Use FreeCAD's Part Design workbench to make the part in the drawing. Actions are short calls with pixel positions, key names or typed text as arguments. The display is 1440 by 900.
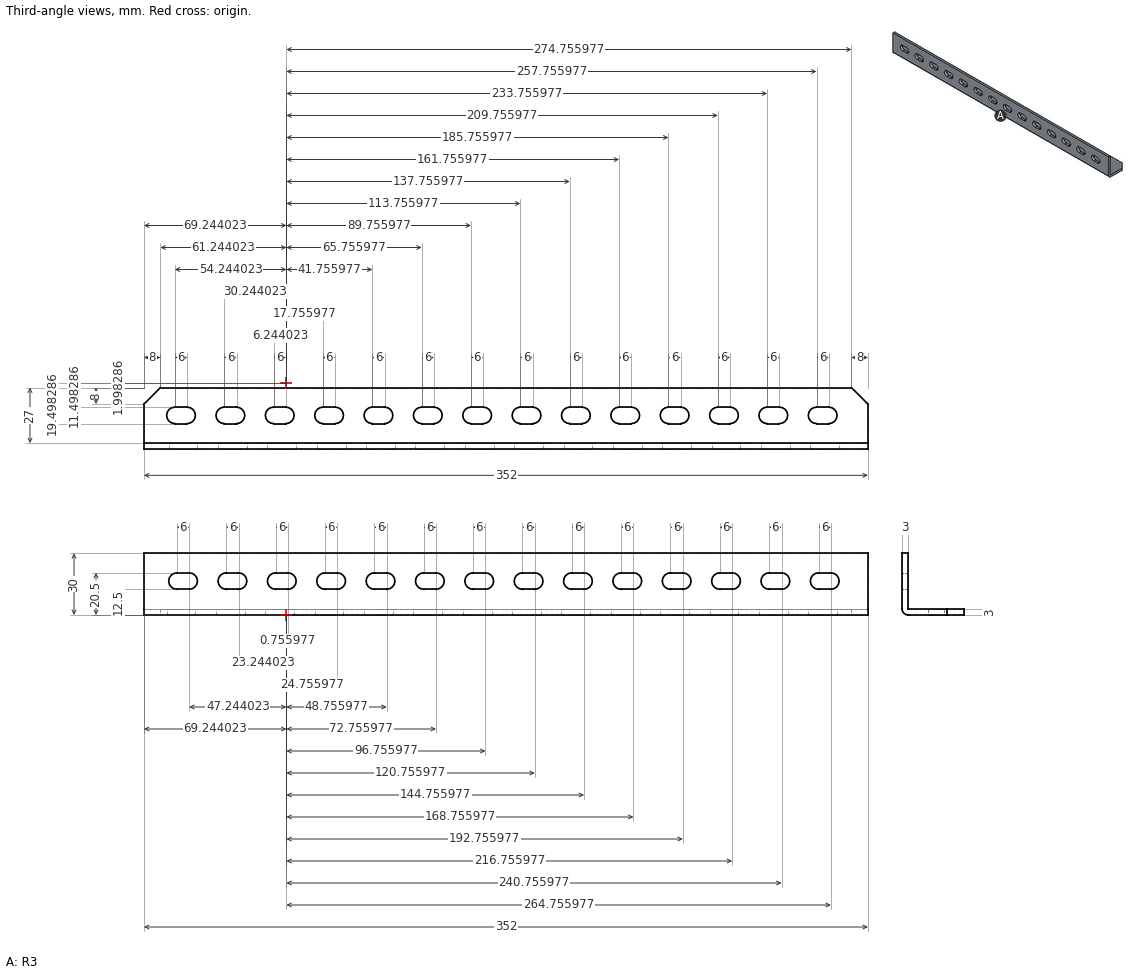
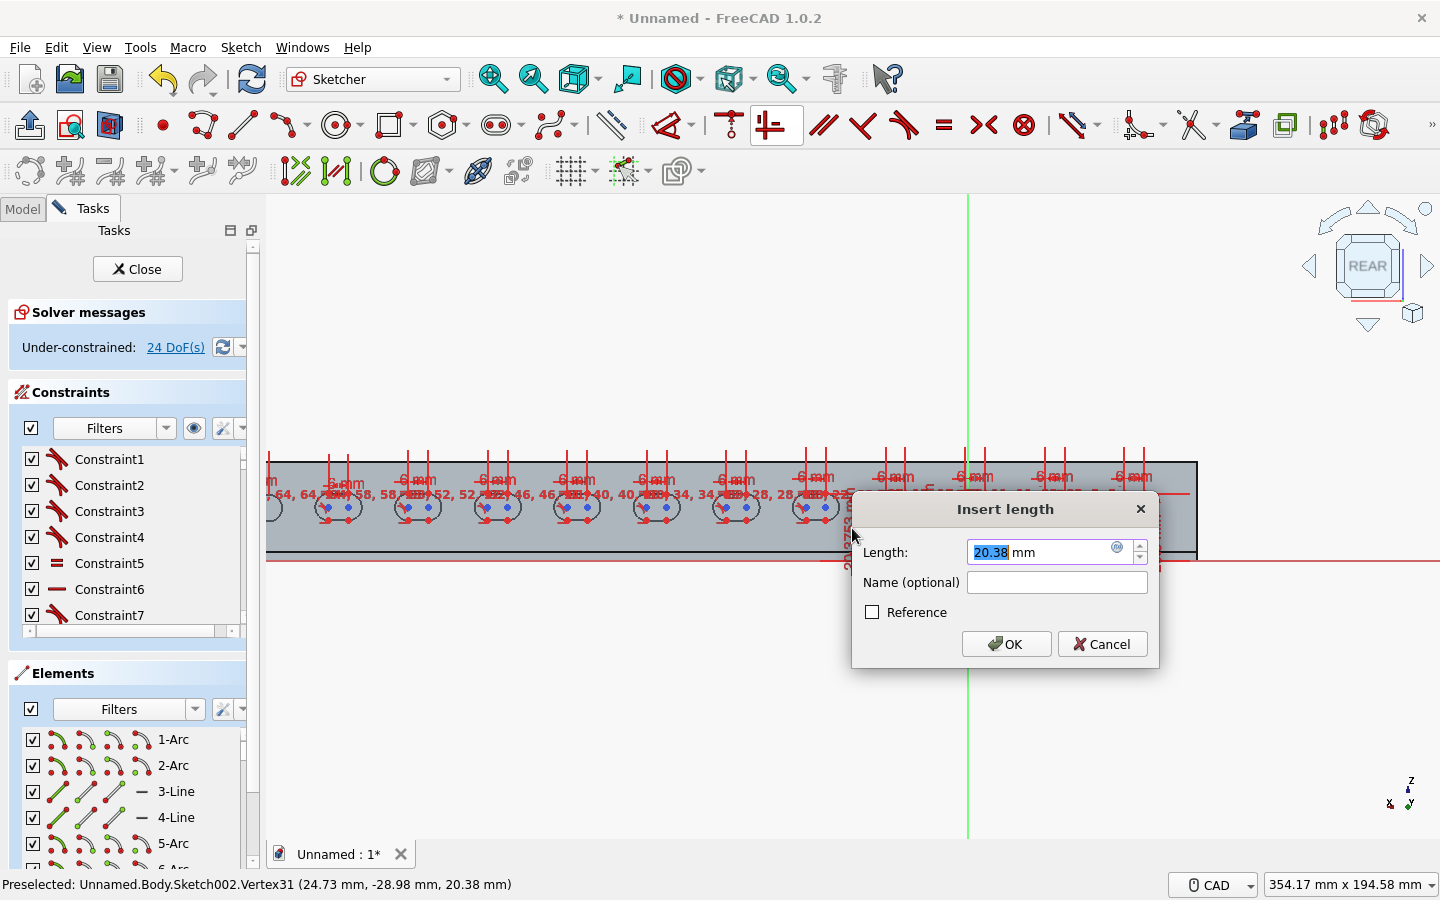
text(20.5)
key(Return)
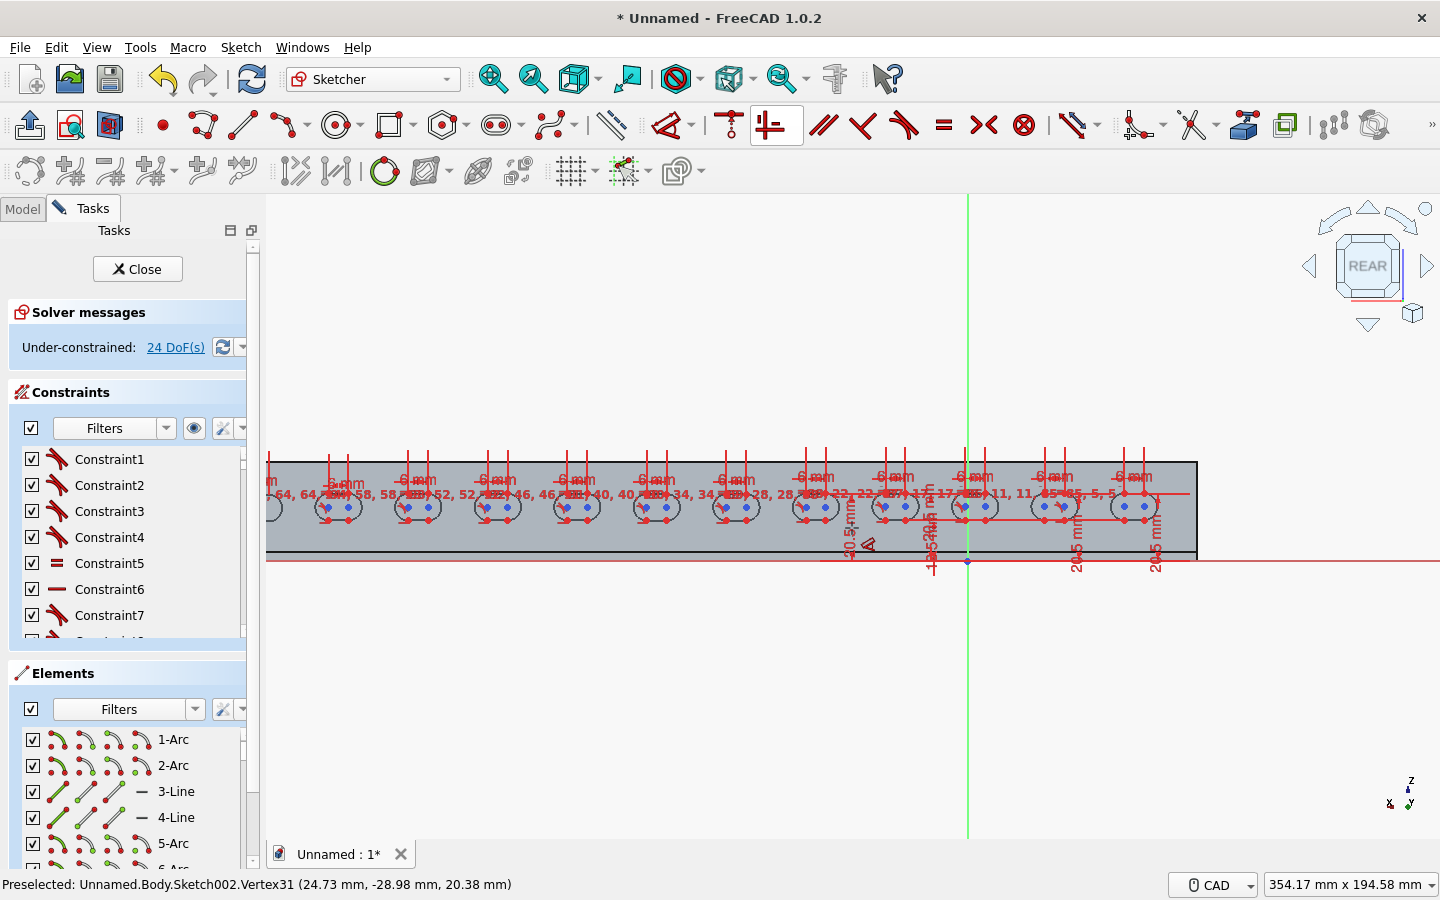
click(806, 494)
click(772, 528)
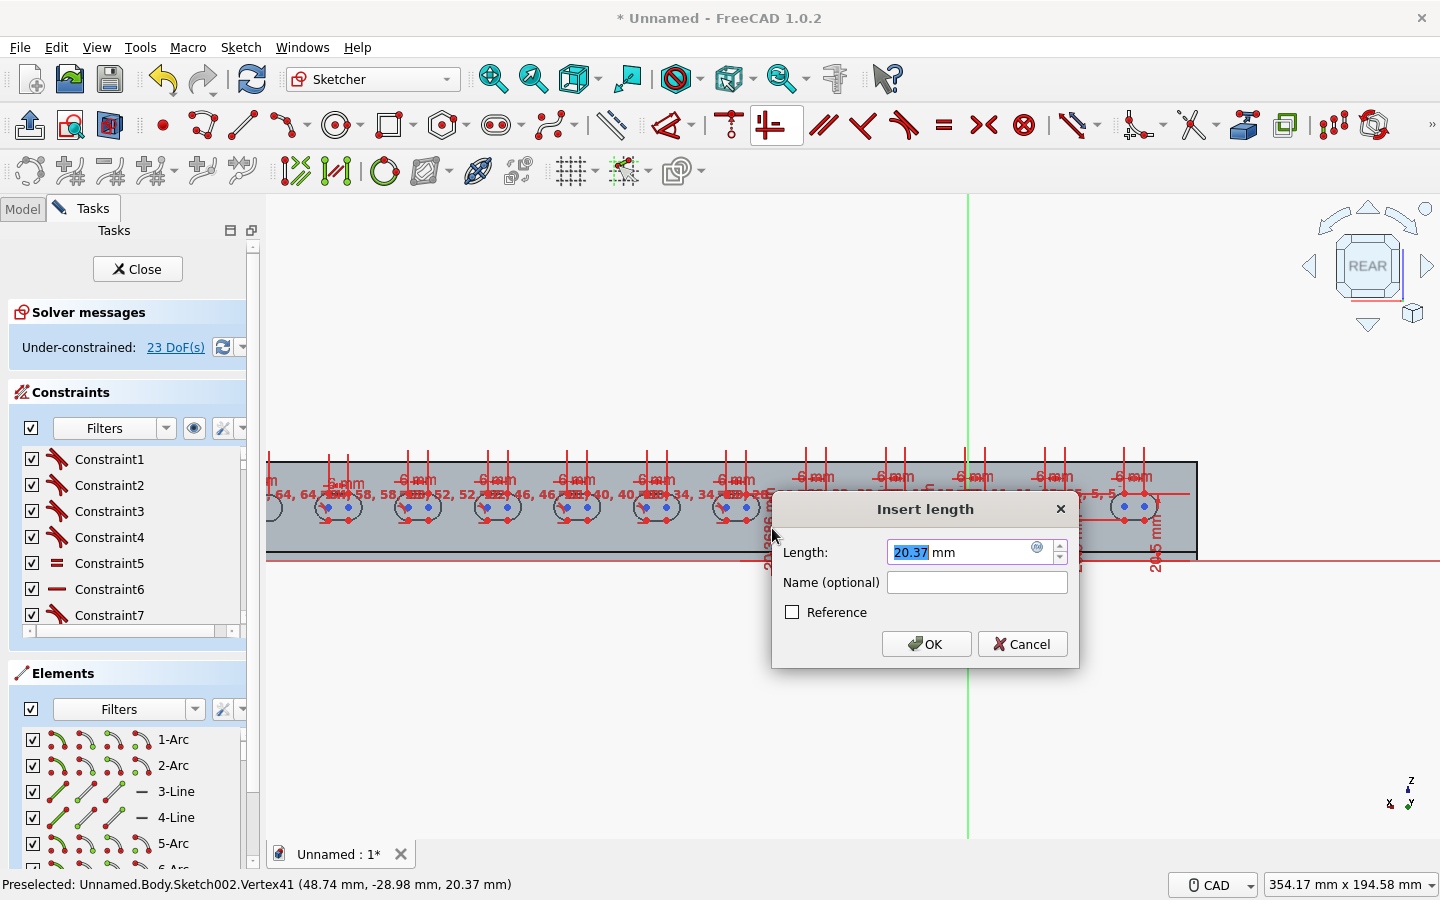
text(20.5)
key(Return)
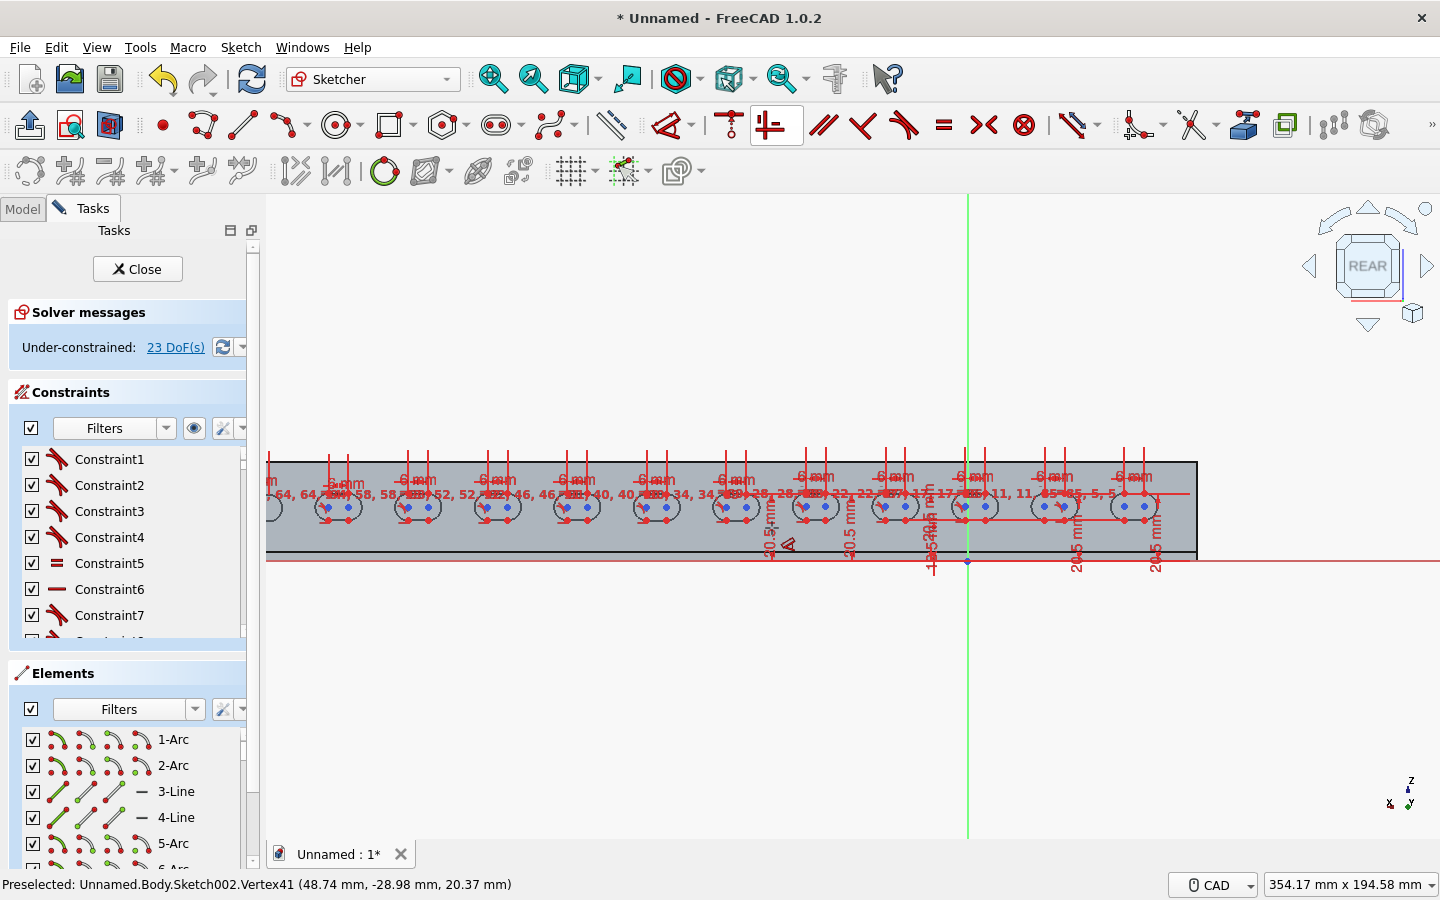
click(726, 494)
click(692, 528)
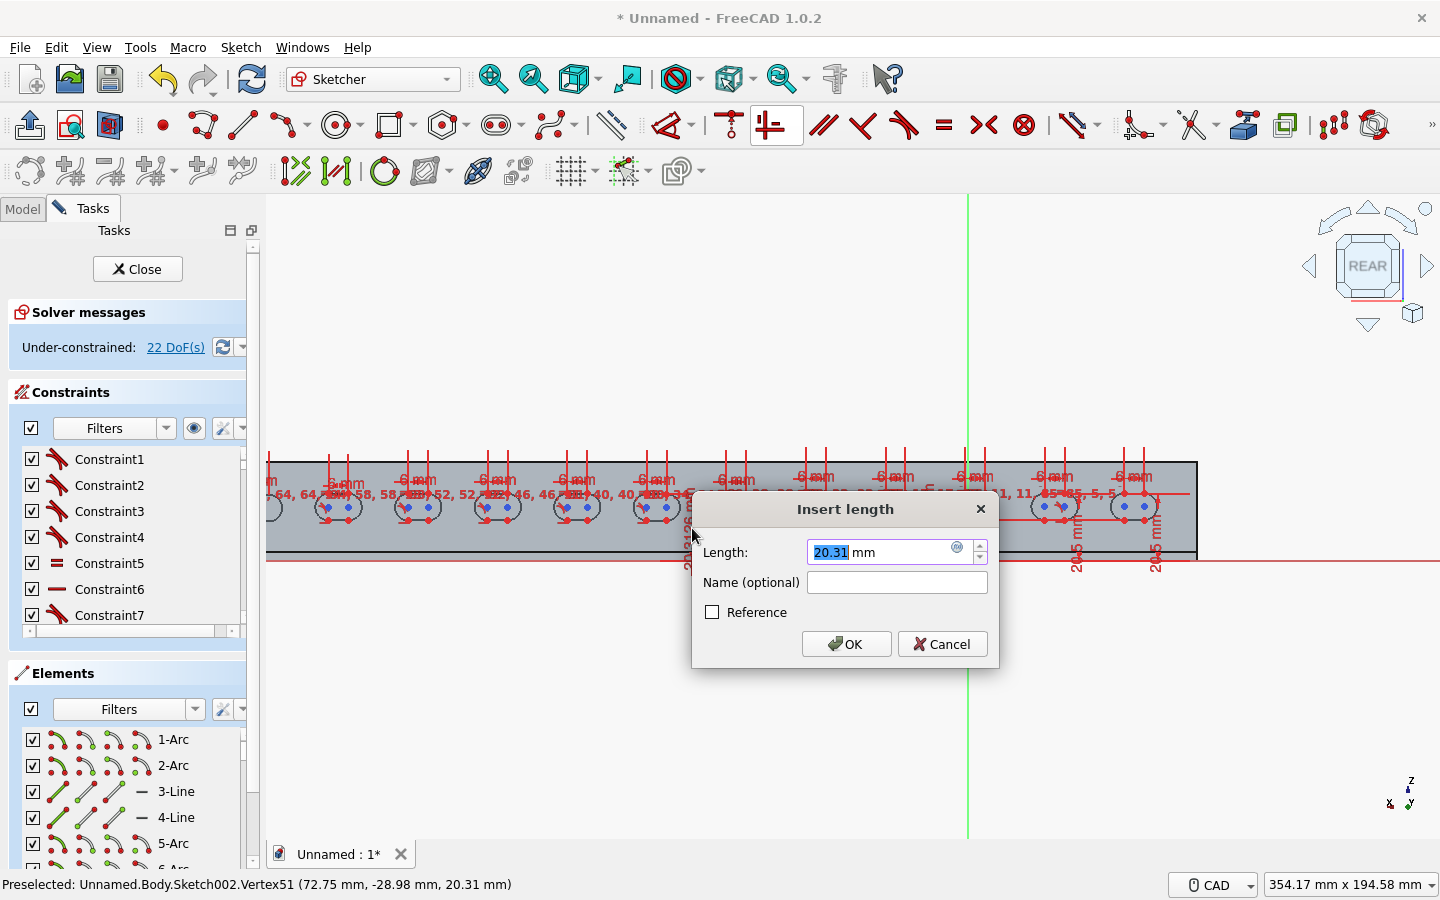
text(20.5)
key(Return)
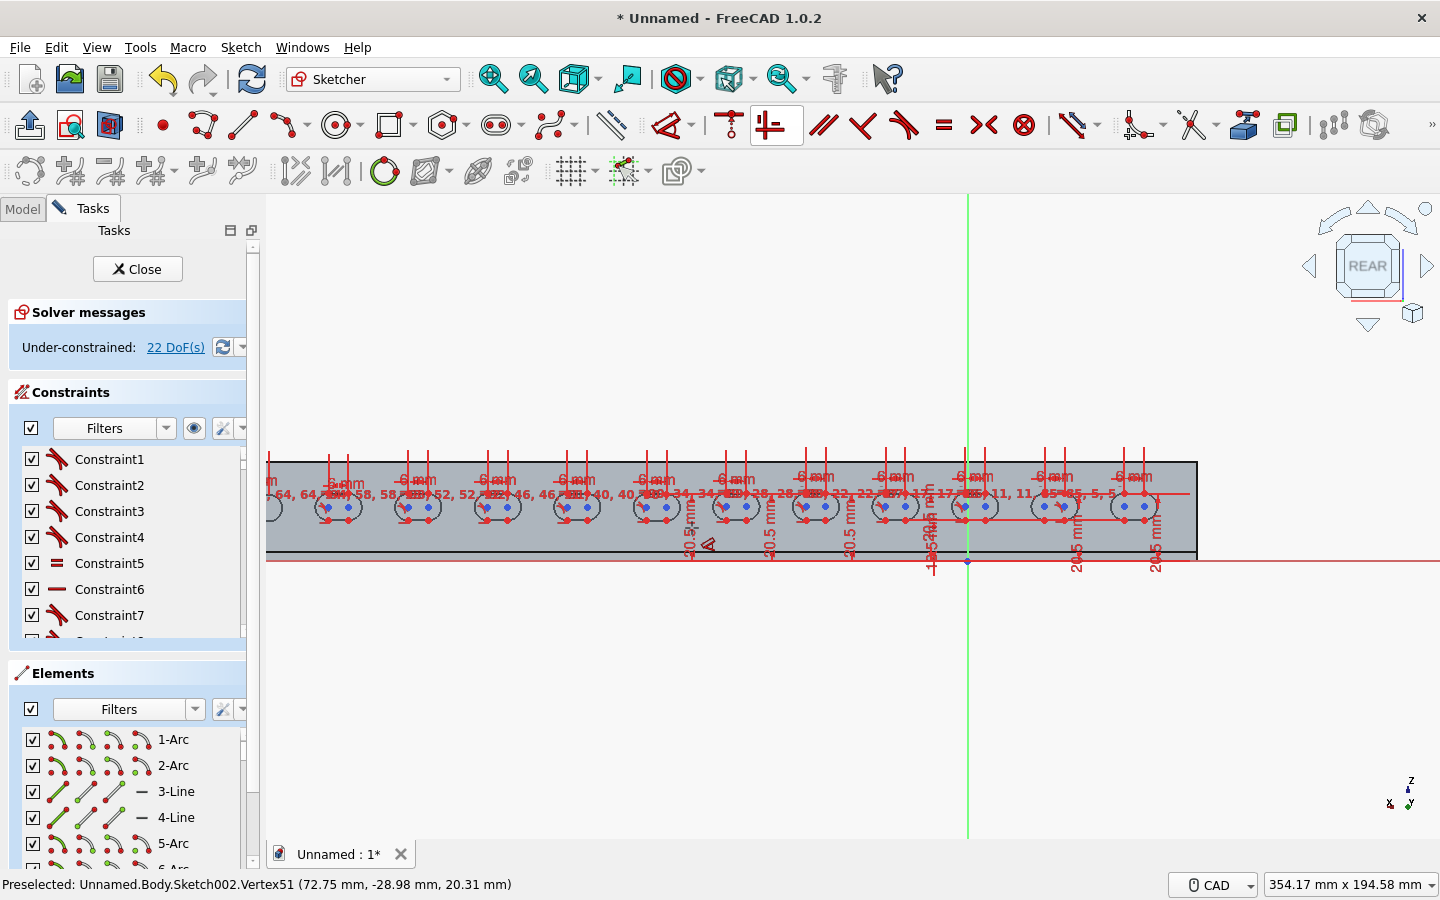
click(647, 494)
click(613, 528)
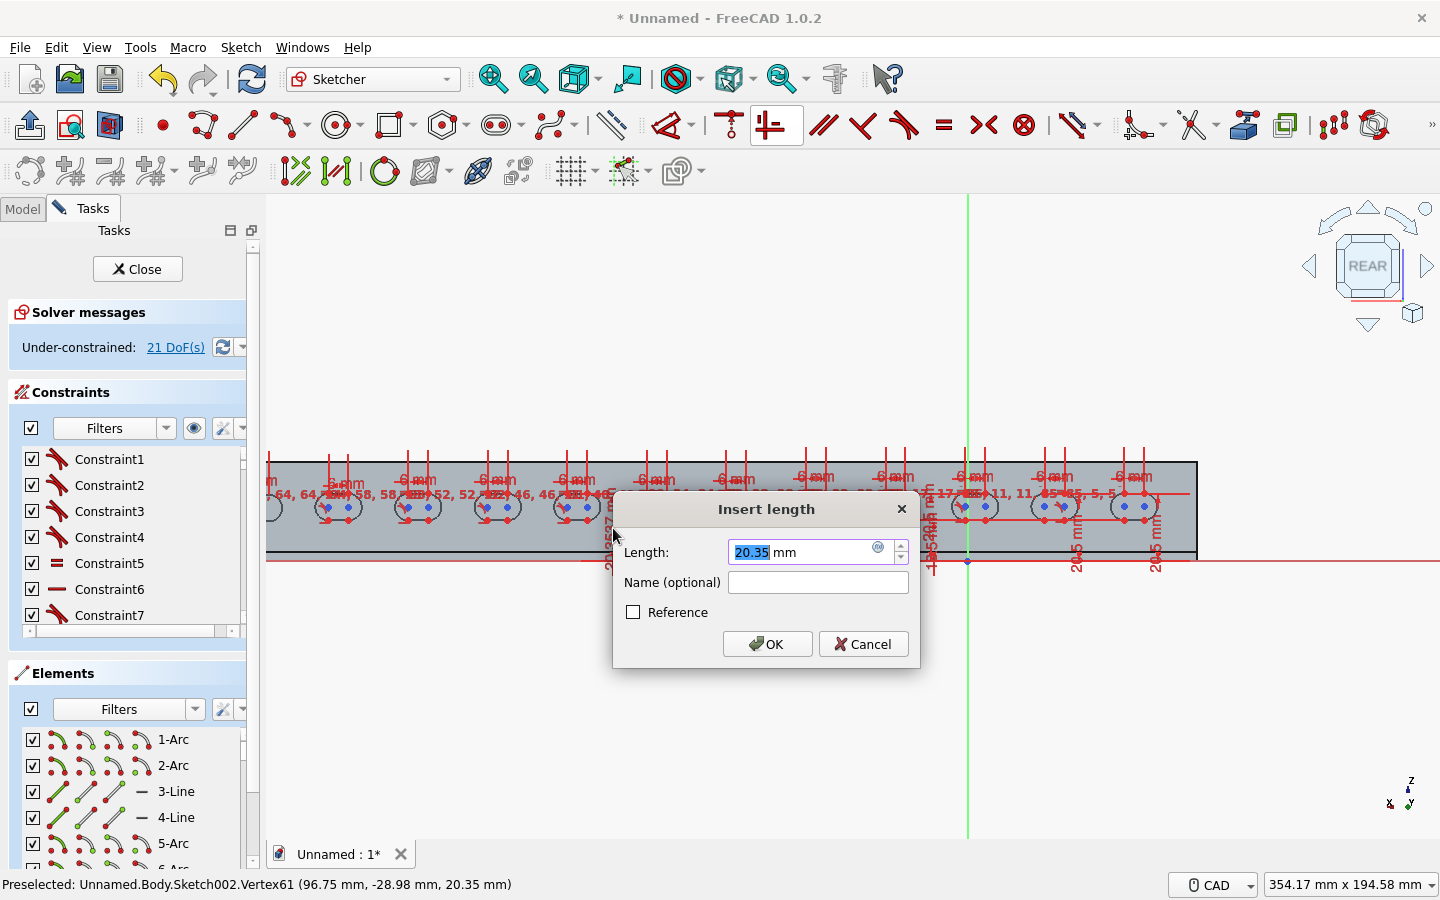
text(20.5)
key(Return)